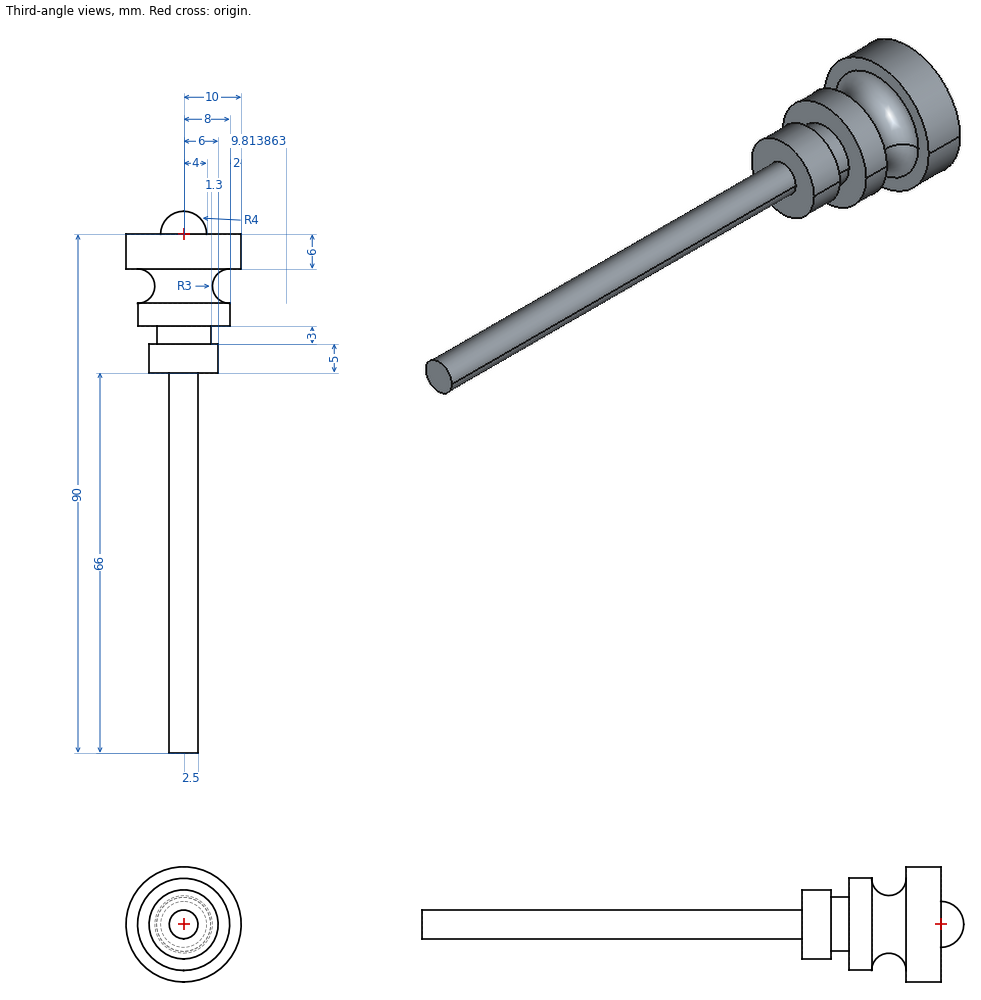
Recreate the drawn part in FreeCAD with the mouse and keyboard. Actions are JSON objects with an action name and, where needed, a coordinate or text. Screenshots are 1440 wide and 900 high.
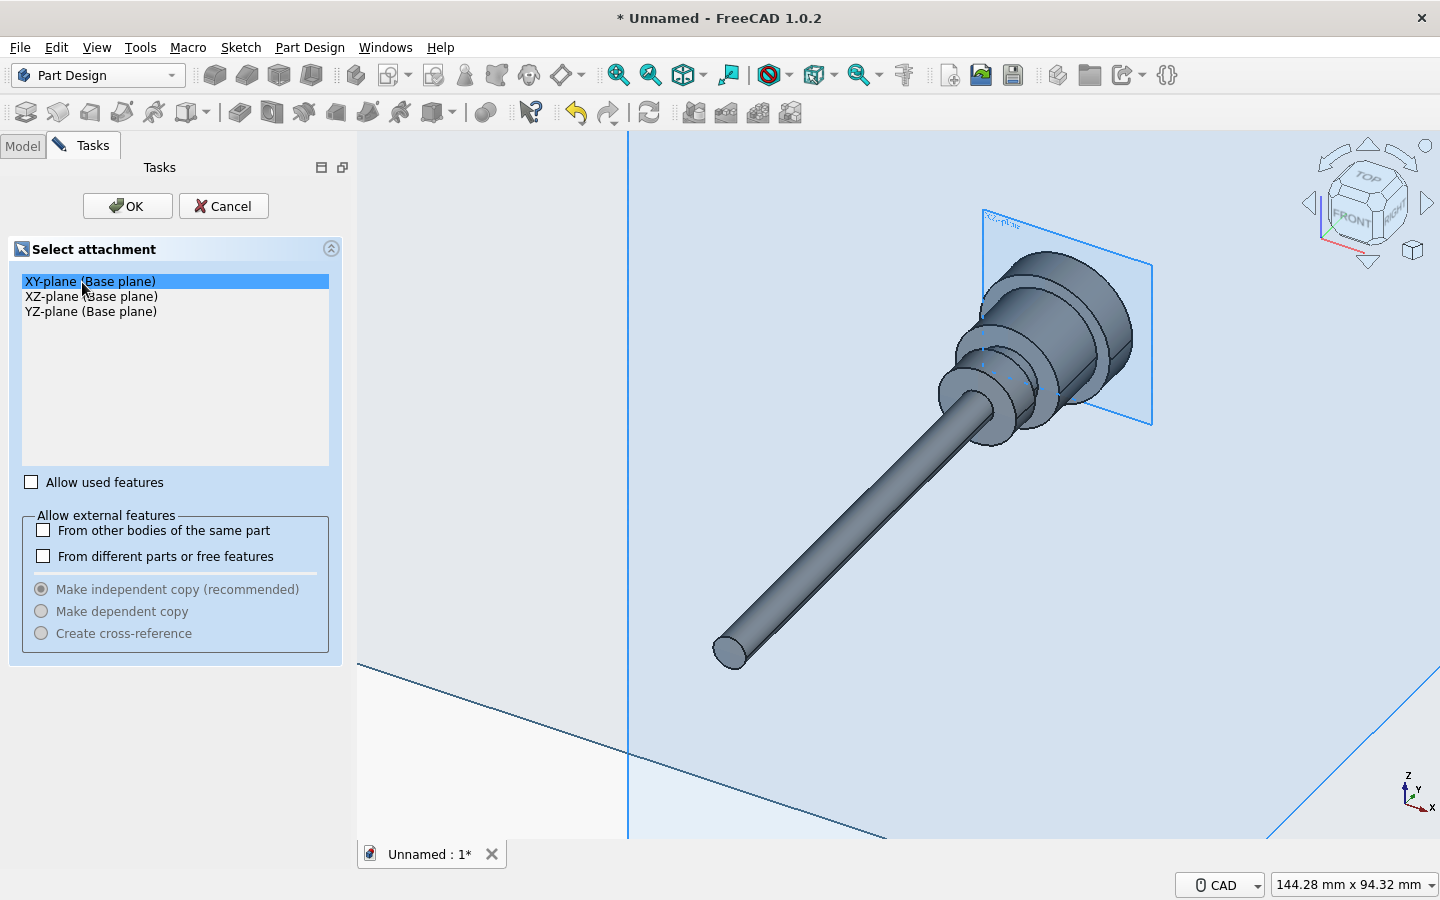
{"action": "left_click", "coordinate": [128, 206]}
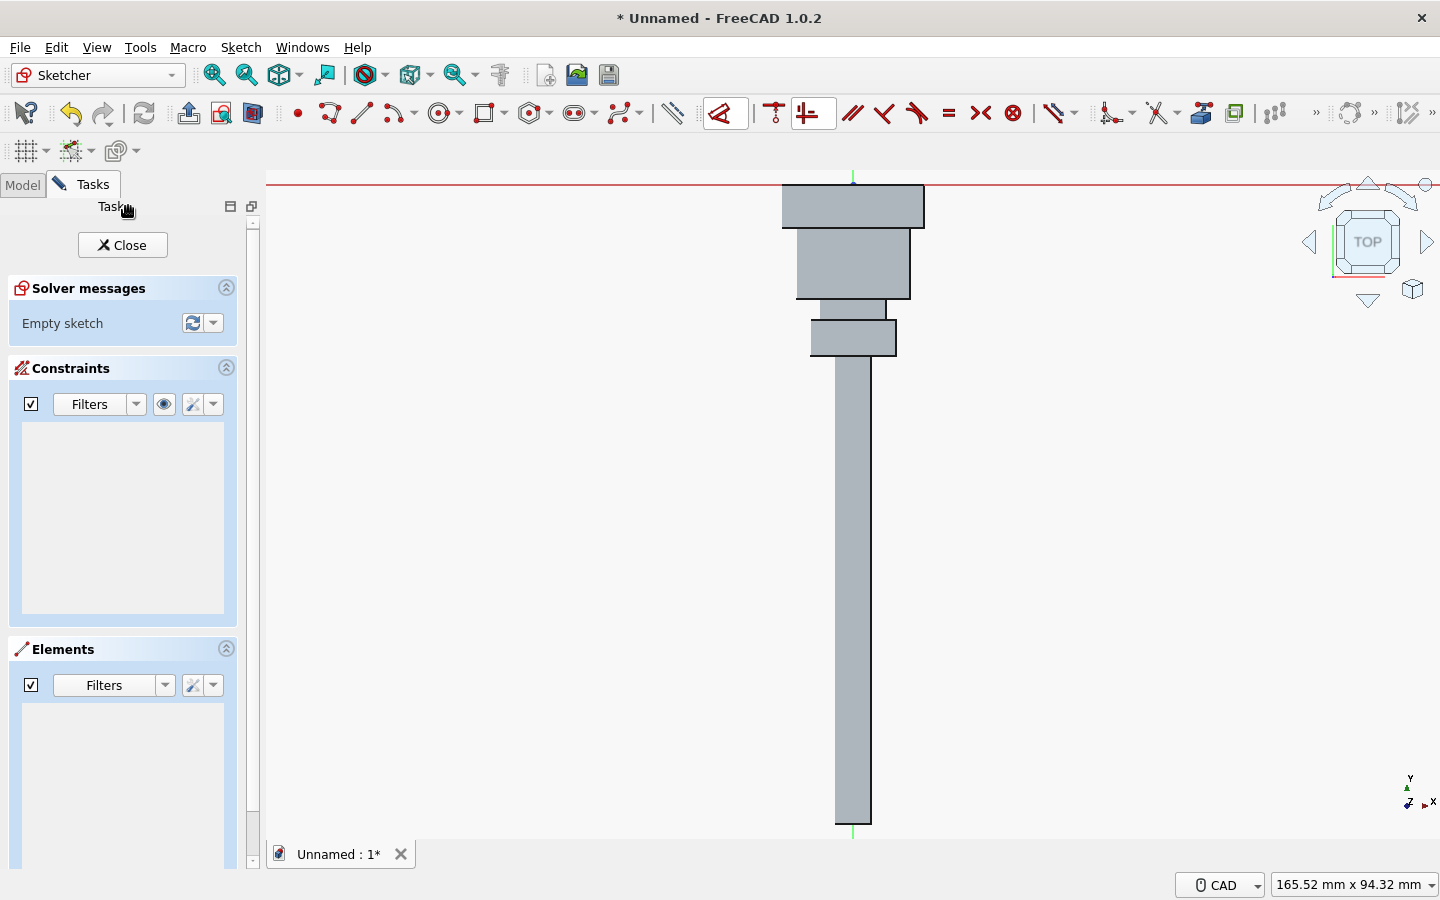
{"action": "left_click", "coordinate": [254, 114]}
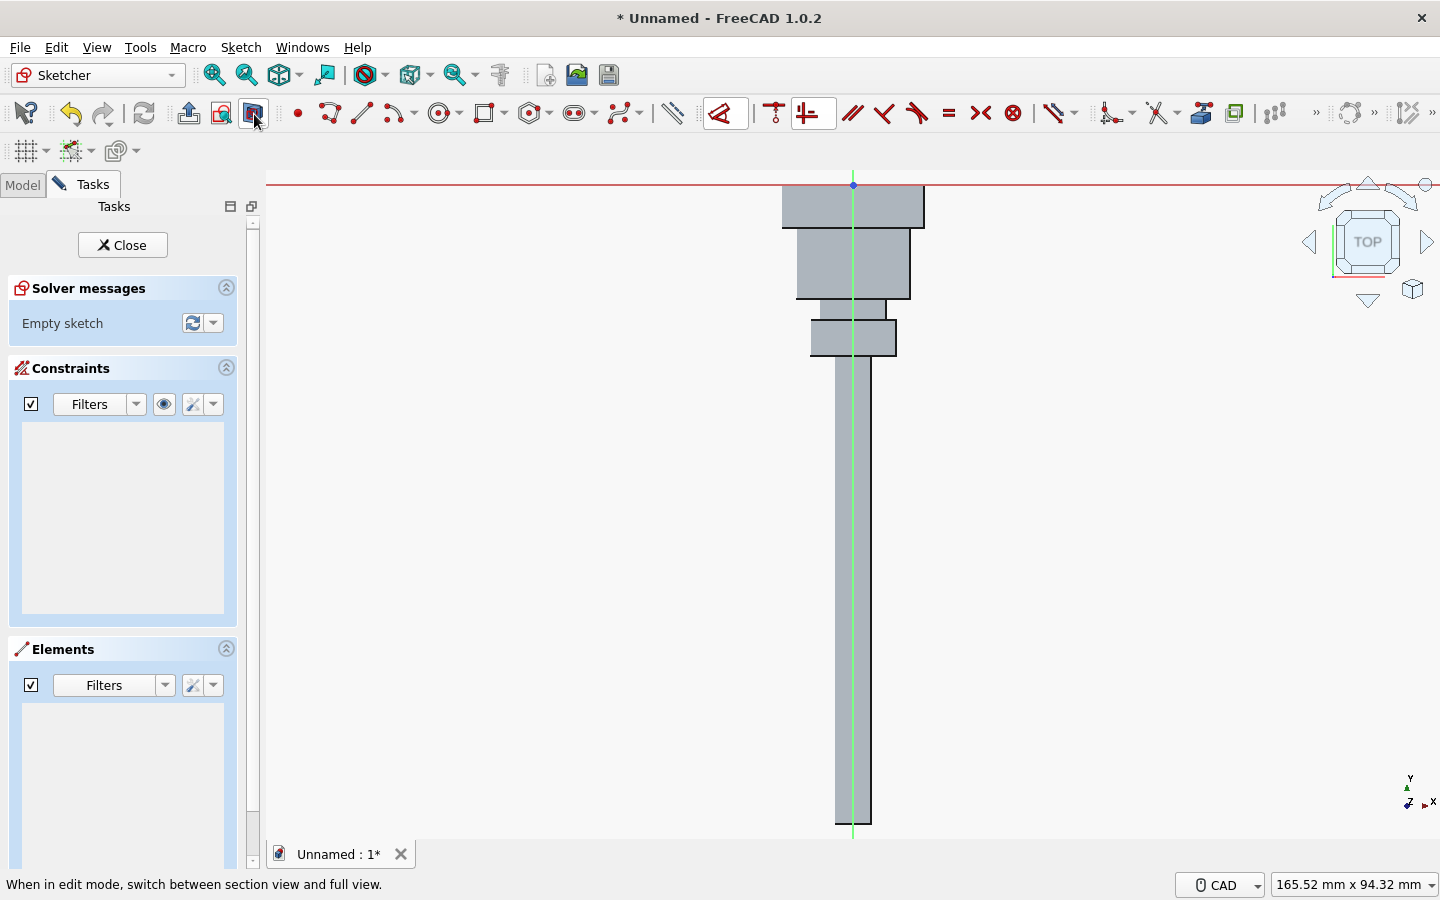
{"action": "scroll", "coordinate": [784, 504], "scroll_direction": "down", "scroll_amount": 5}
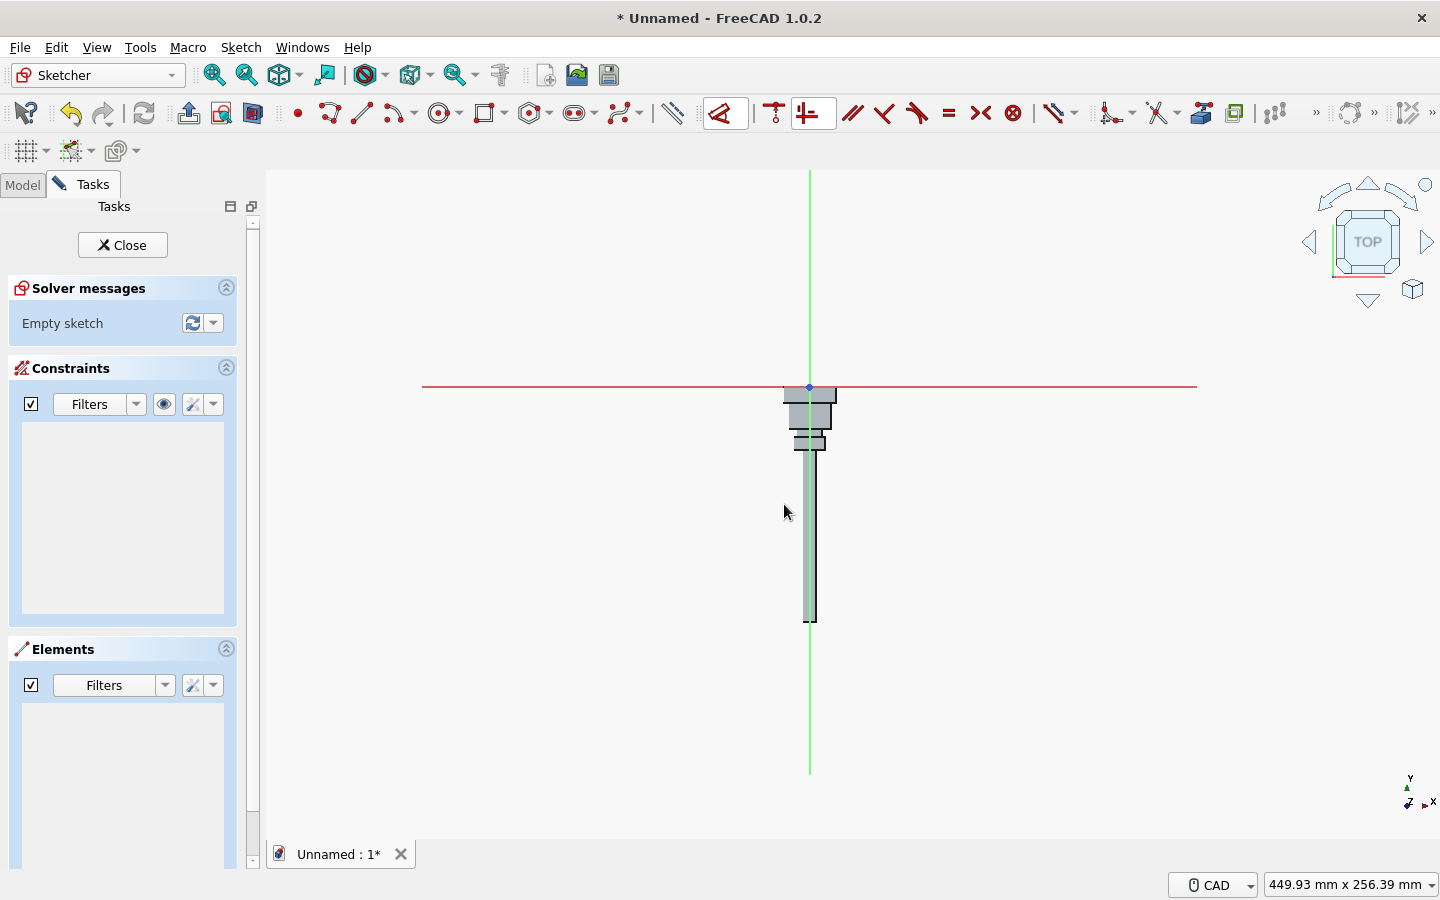
{"action": "scroll", "coordinate": [837, 395], "scroll_direction": "up", "scroll_amount": 13}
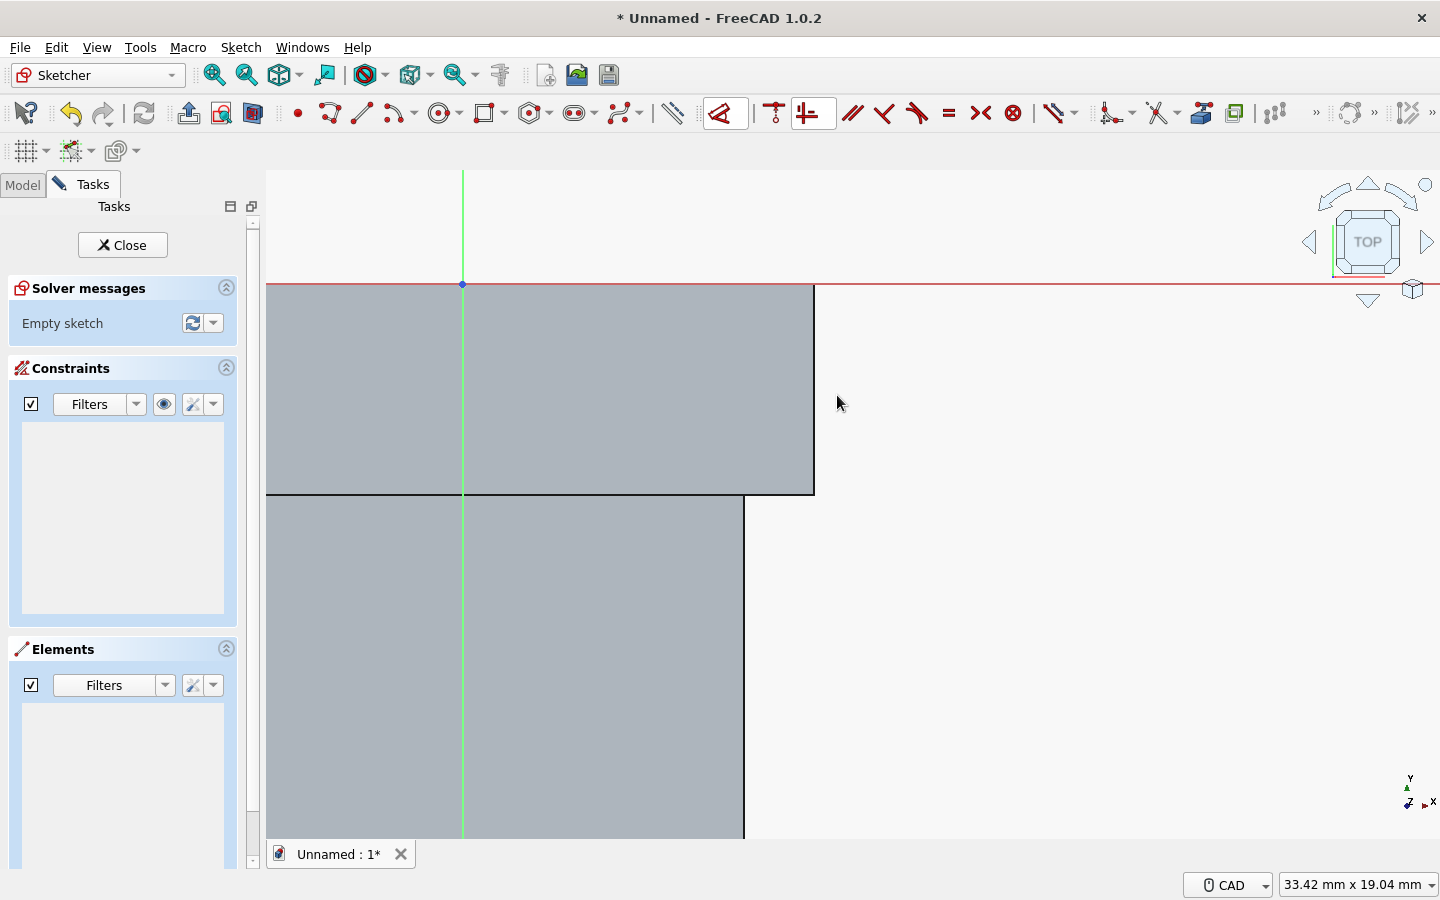
{"action": "key", "text": "g m"}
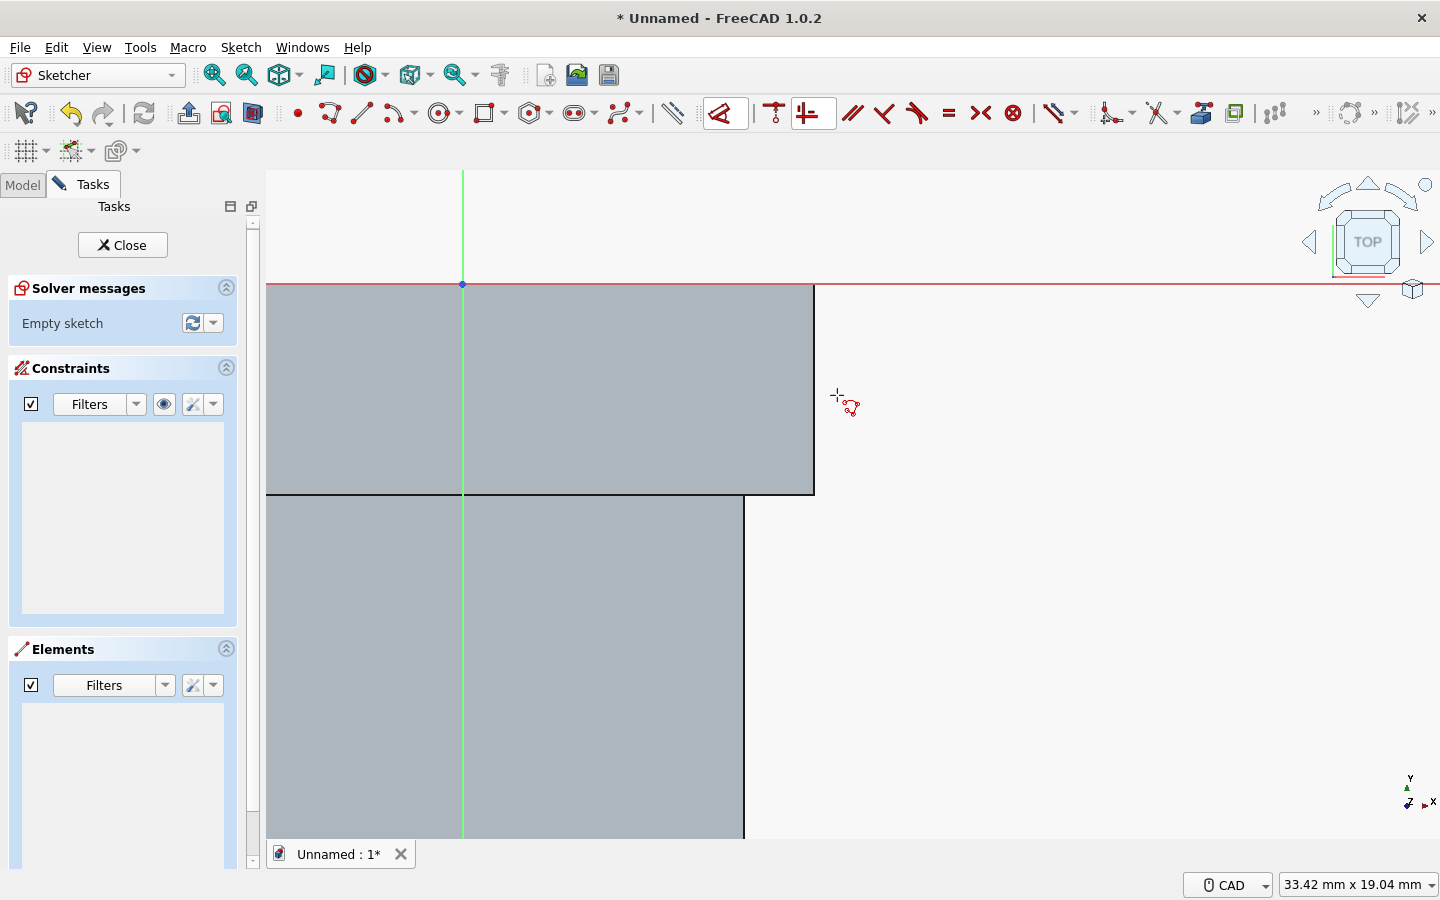
{"action": "left_click", "coordinate": [744, 706]}
{"action": "left_click", "coordinate": [1089, 706]}
{"action": "left_click", "coordinate": [1089, 495]}
{"action": "left_click", "coordinate": [744, 495]}
{"action": "right_click", "coordinate": [744, 495]}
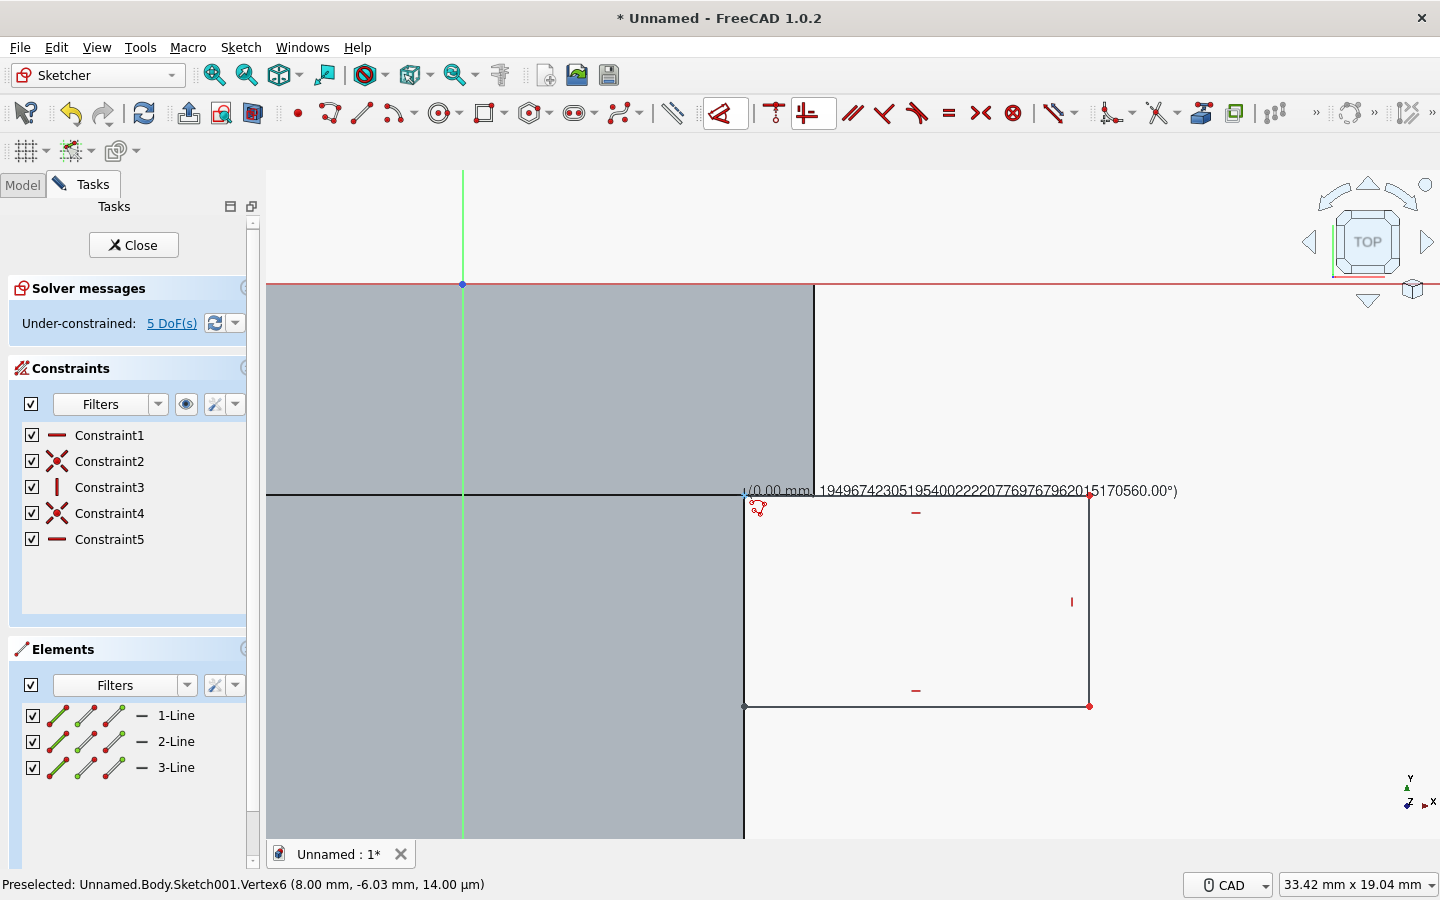
{"action": "key", "text": "g 3 a"}